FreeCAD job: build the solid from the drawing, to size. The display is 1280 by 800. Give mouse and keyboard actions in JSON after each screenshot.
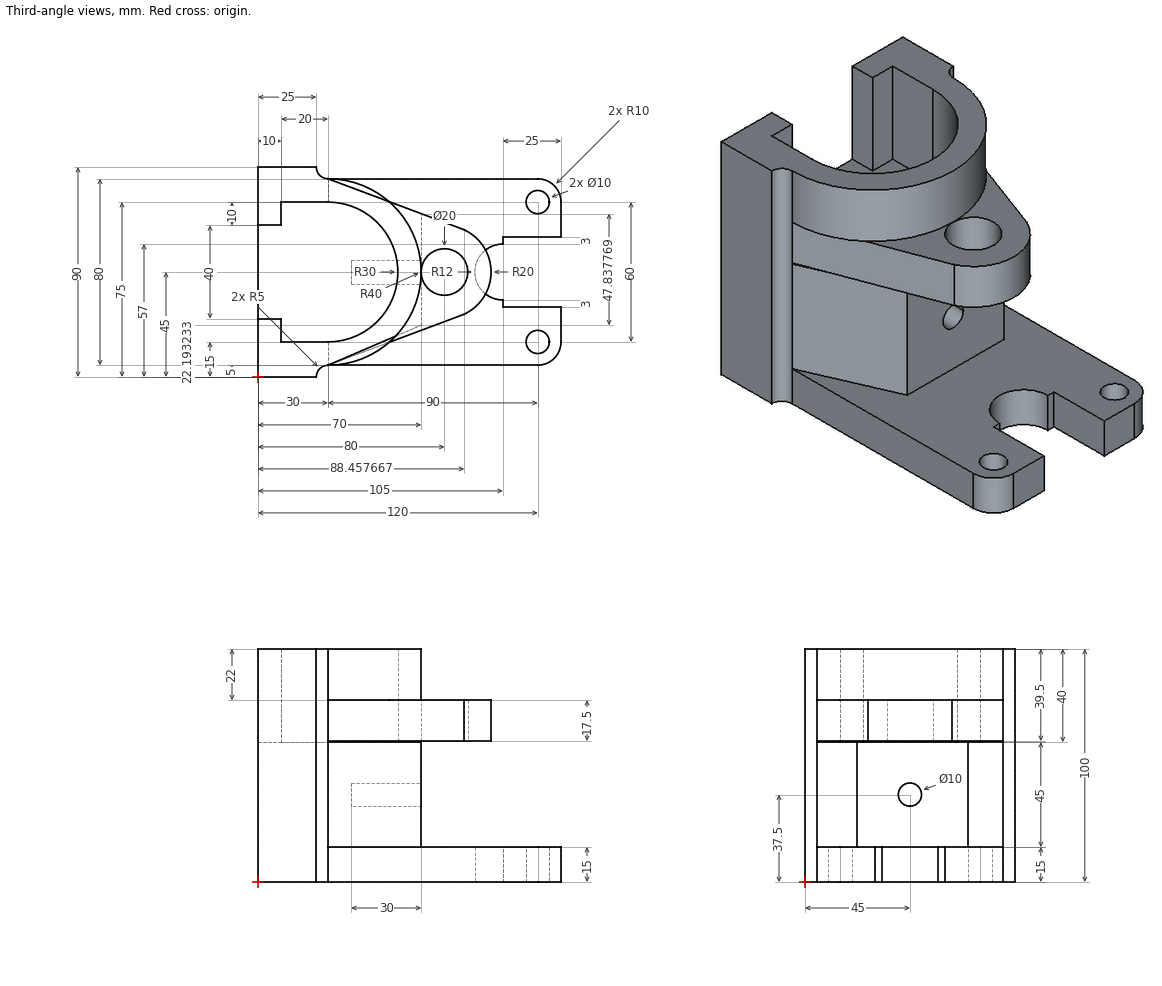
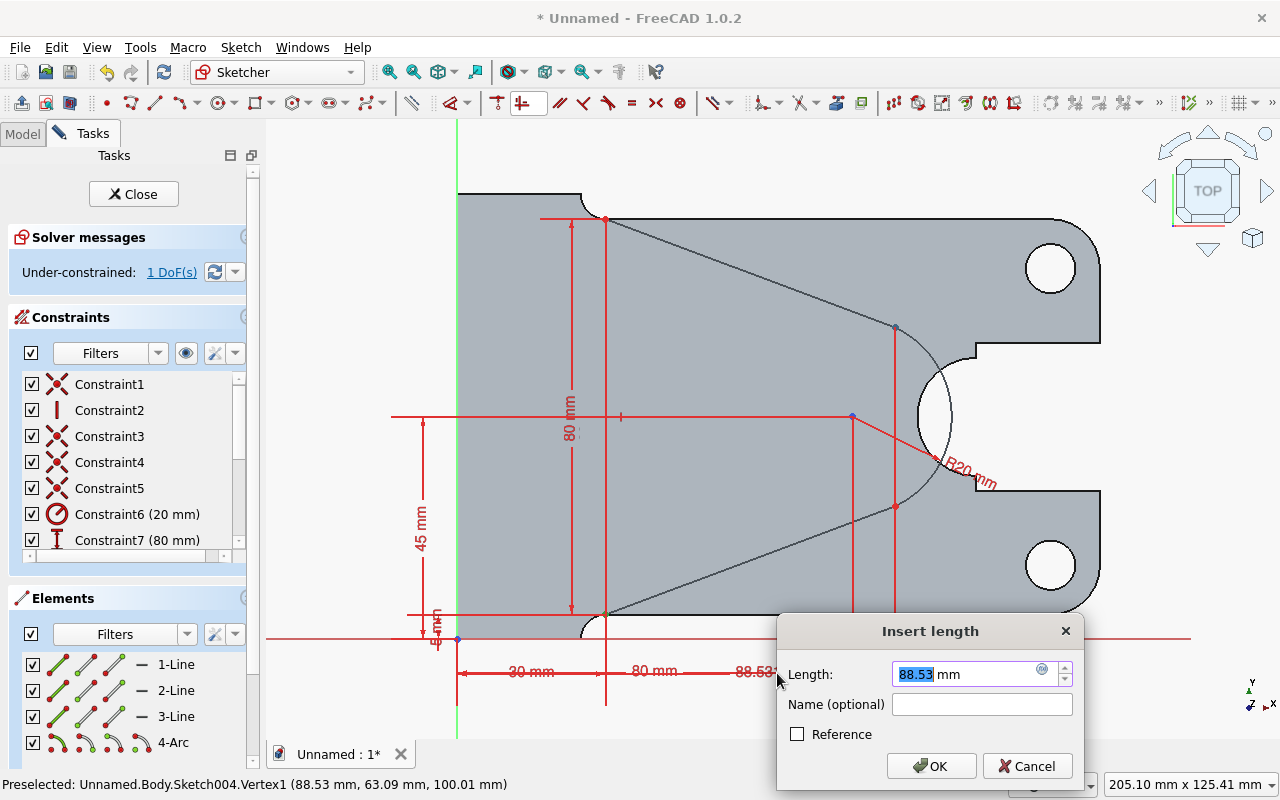
{"action": "type", "text": "88.457667"}
{"action": "key", "text": "Return"}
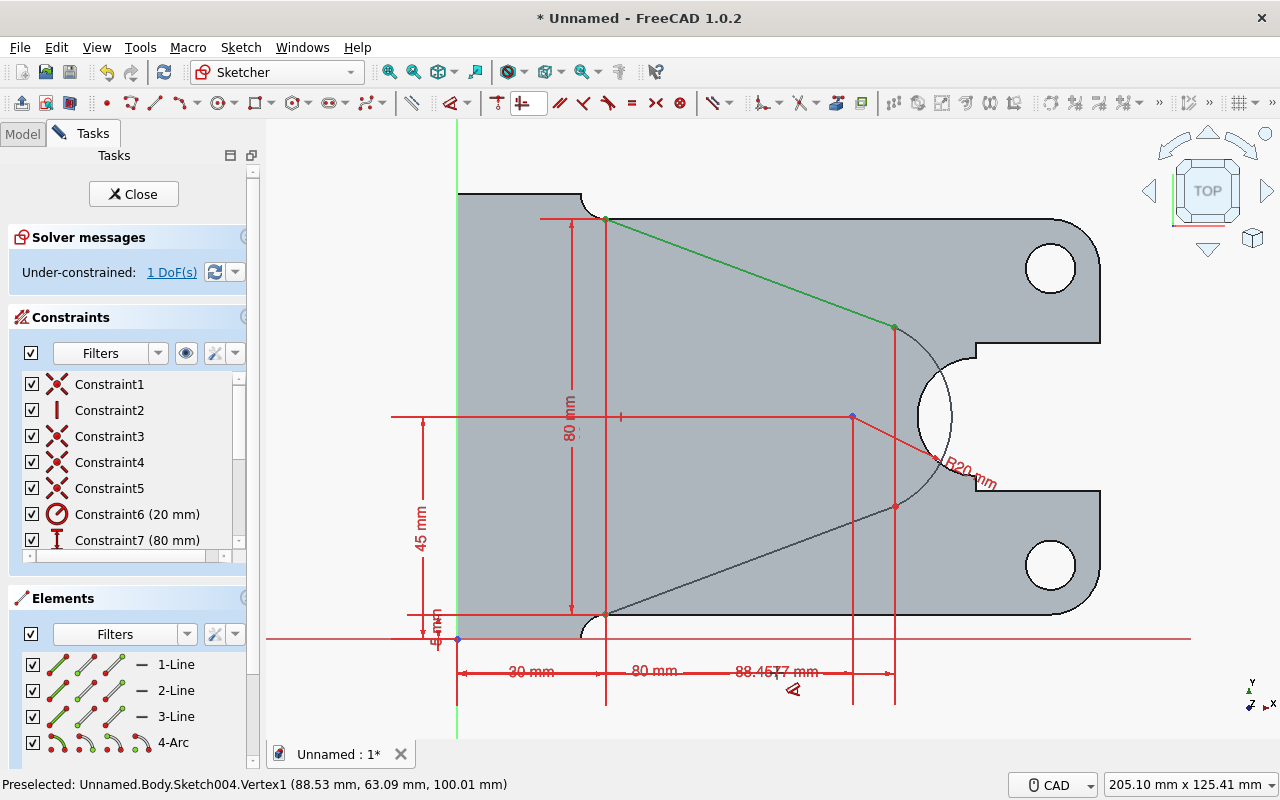
{"action": "left_click", "coordinate": [895, 506]}
{"action": "left_click", "coordinate": [676, 472]}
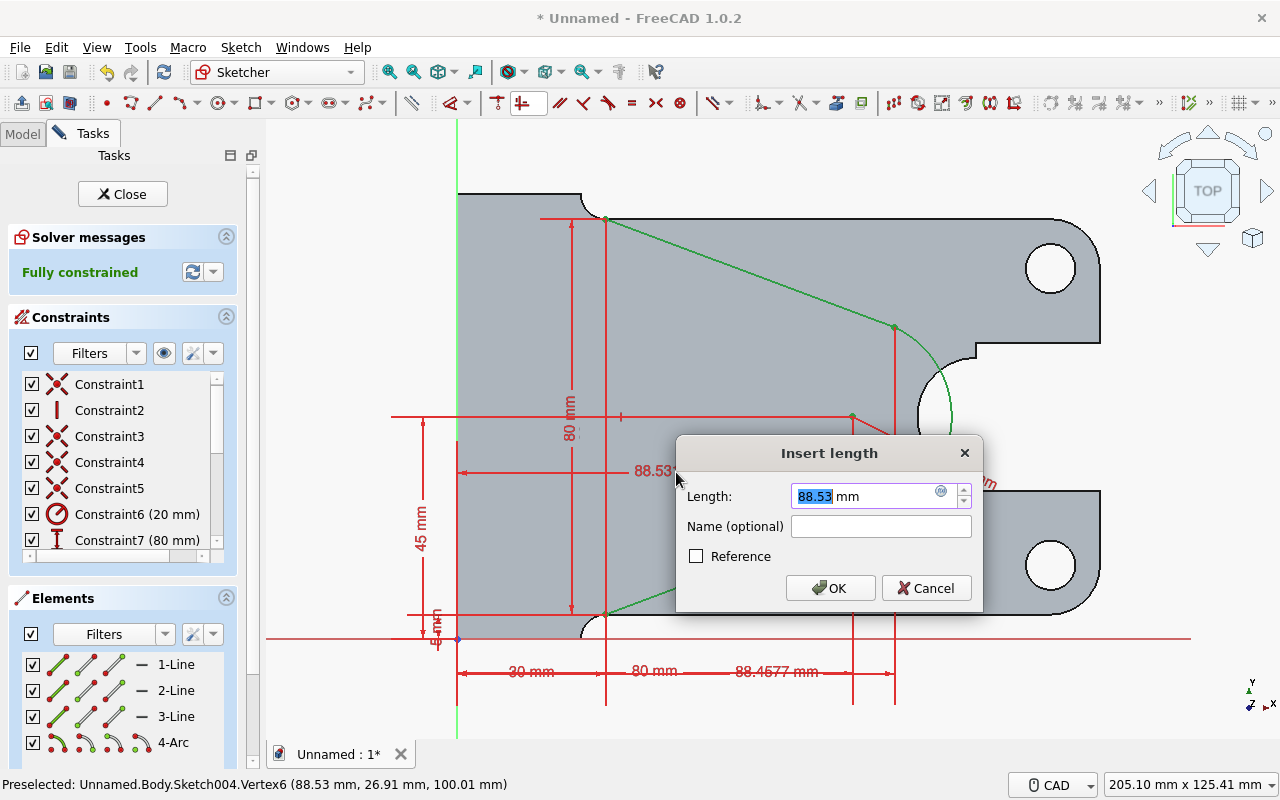
{"action": "type", "text": "88.457667"}
{"action": "key", "text": "Return"}
{"action": "key", "text": "Escape"}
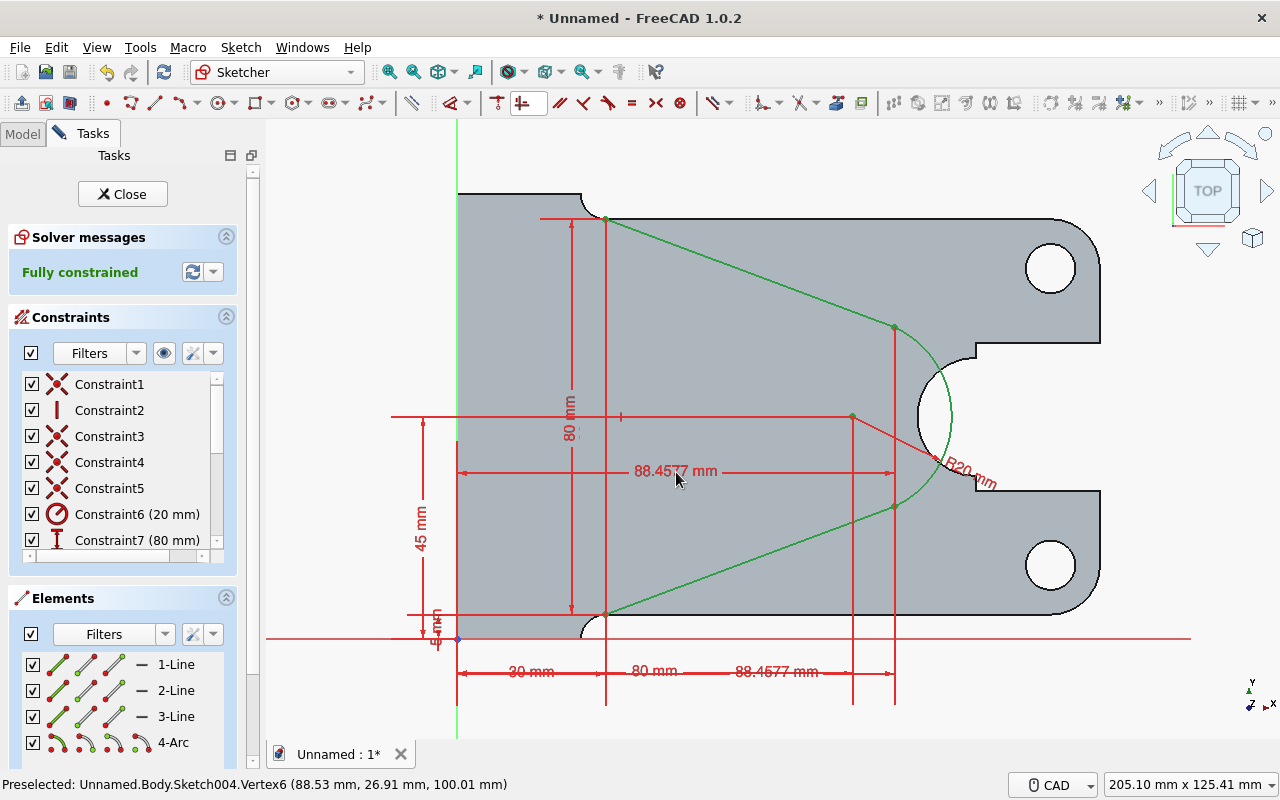
{"action": "left_click", "coordinate": [123, 194]}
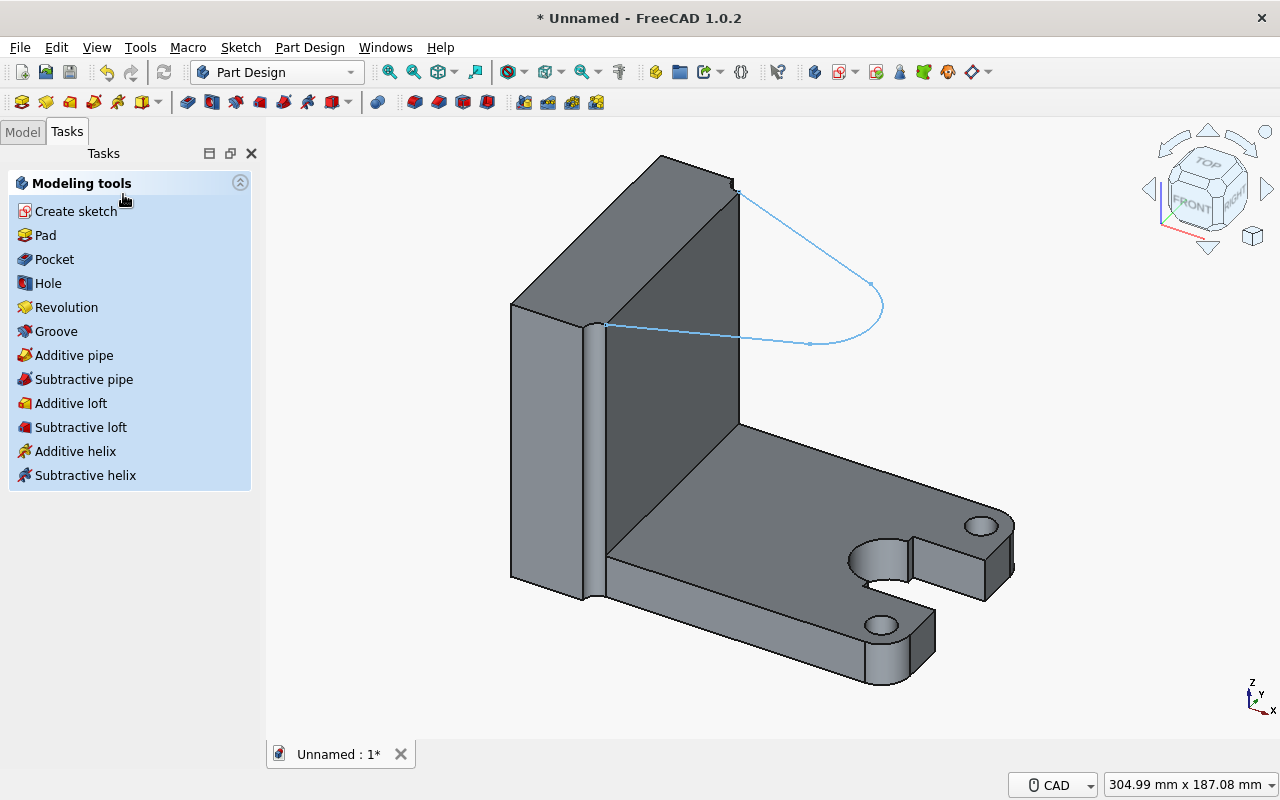
{"action": "left_click", "coordinate": [22, 102]}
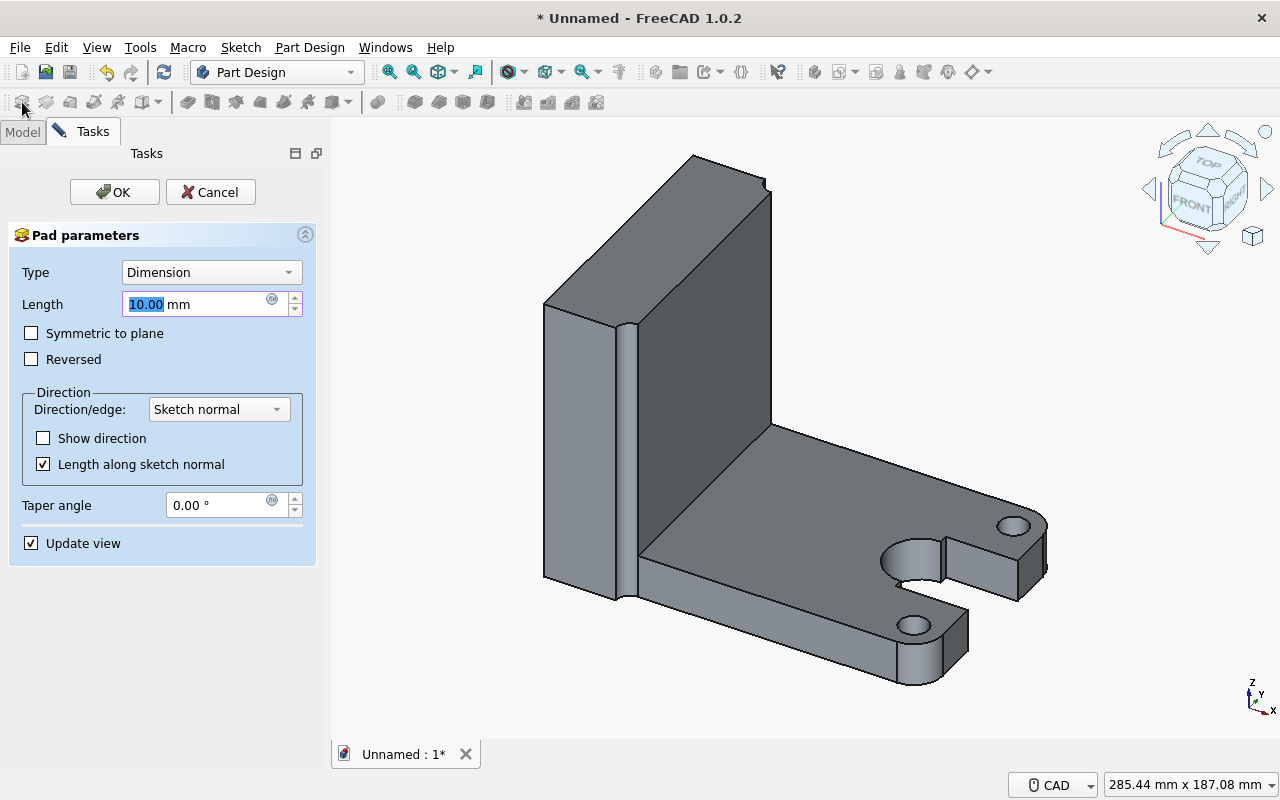
{"action": "type", "text": "39.5"}
{"action": "key", "text": "Tab"}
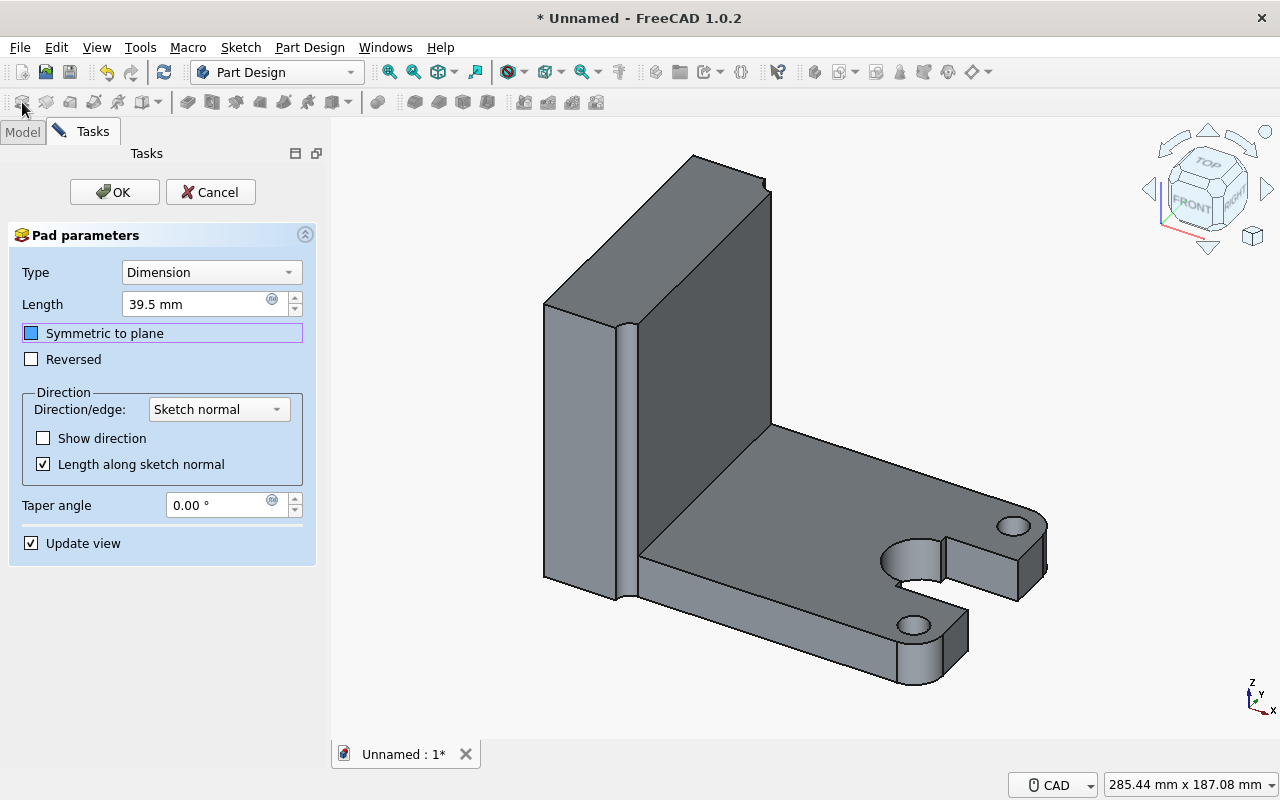
{"action": "left_click", "coordinate": [30, 359]}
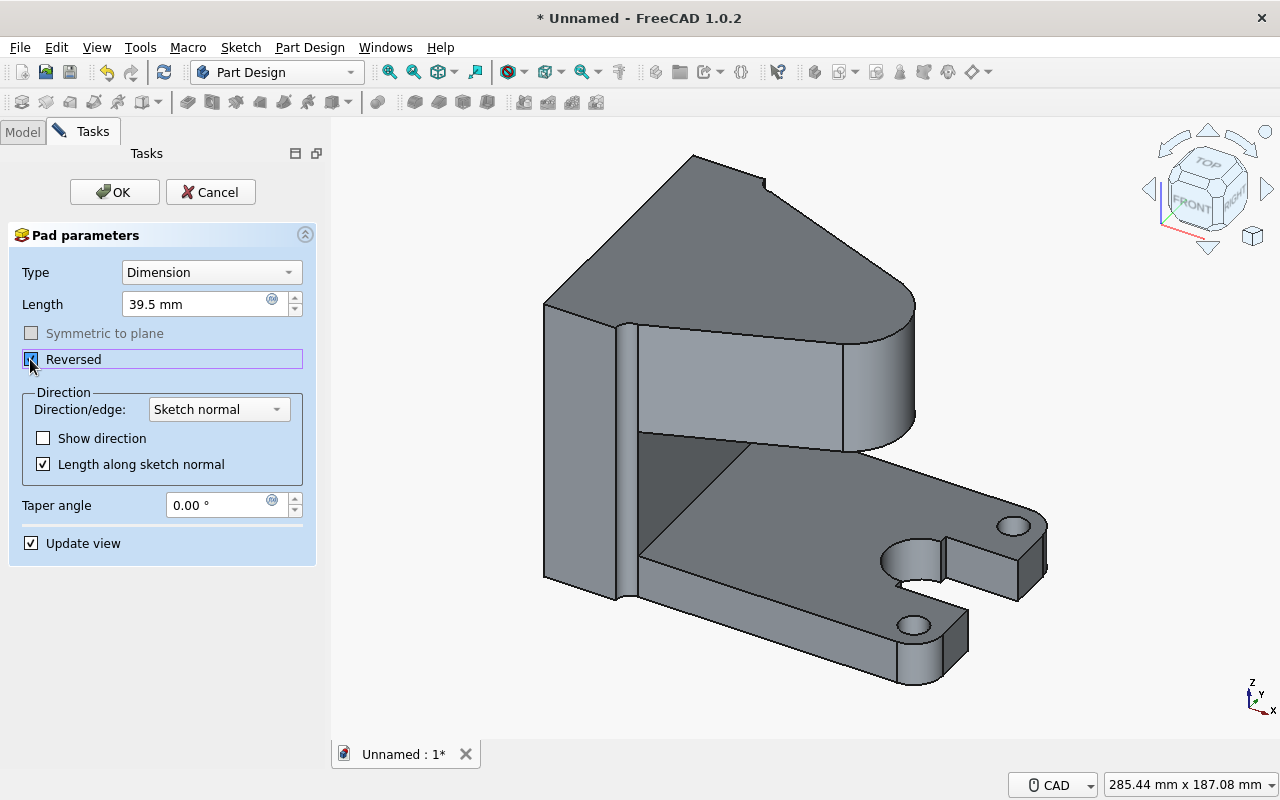
{"action": "left_click", "coordinate": [115, 192]}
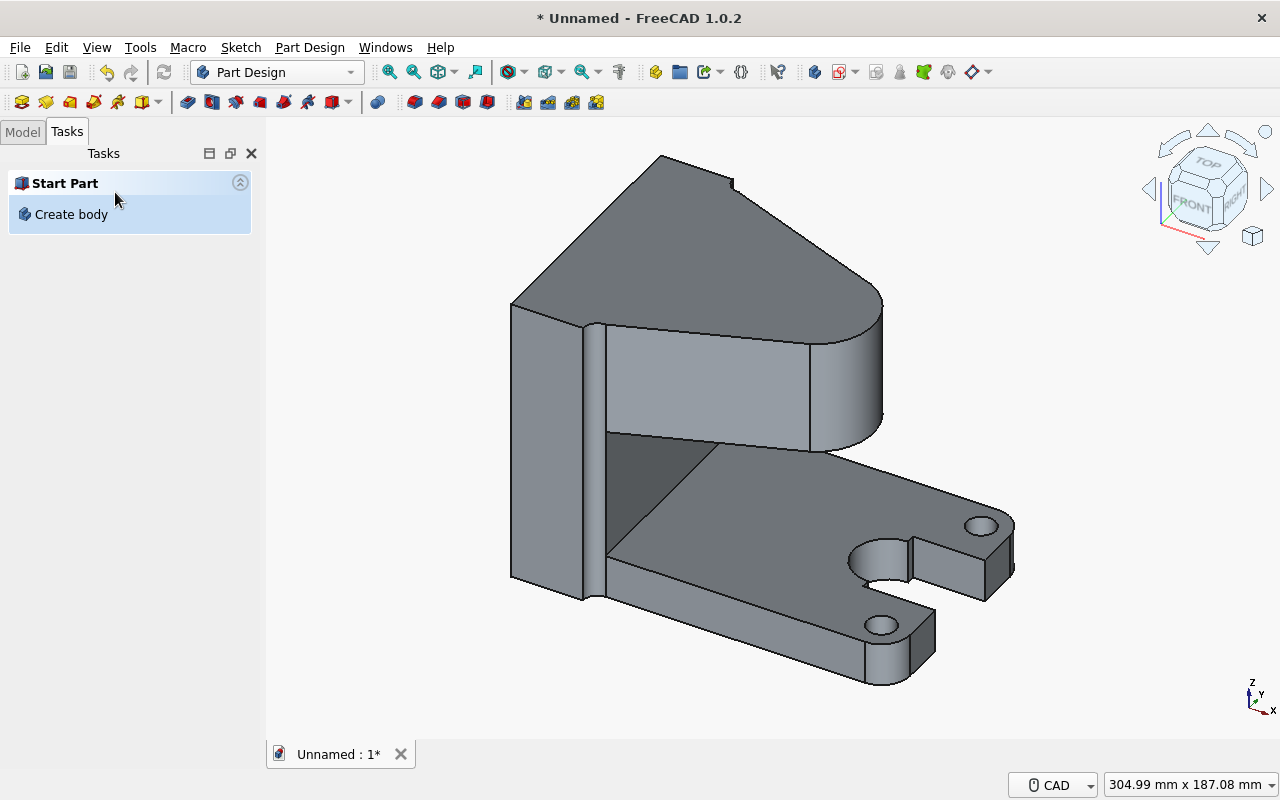
{"action": "left_click", "coordinate": [689, 263]}